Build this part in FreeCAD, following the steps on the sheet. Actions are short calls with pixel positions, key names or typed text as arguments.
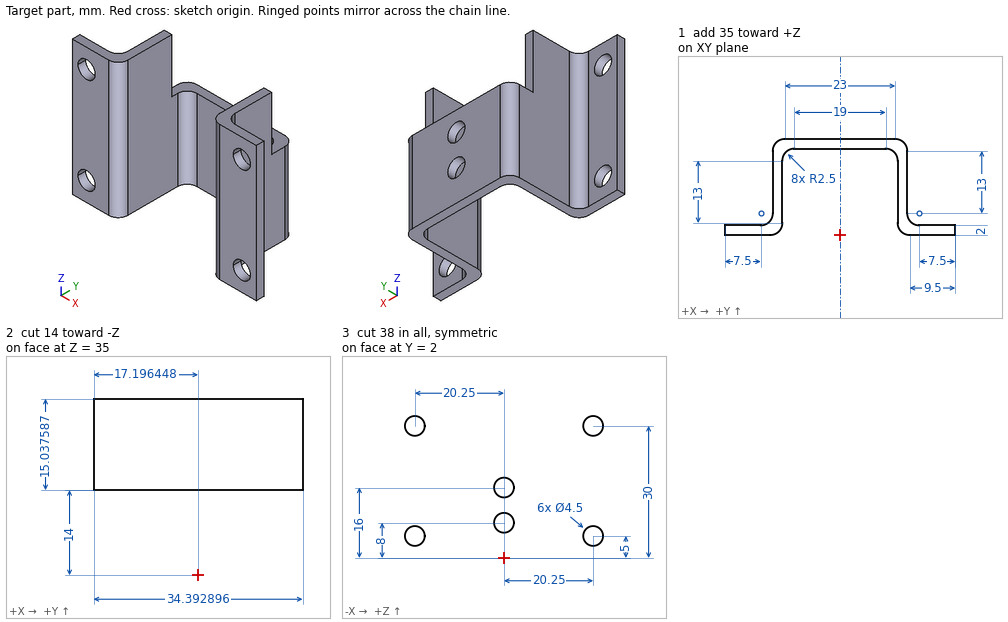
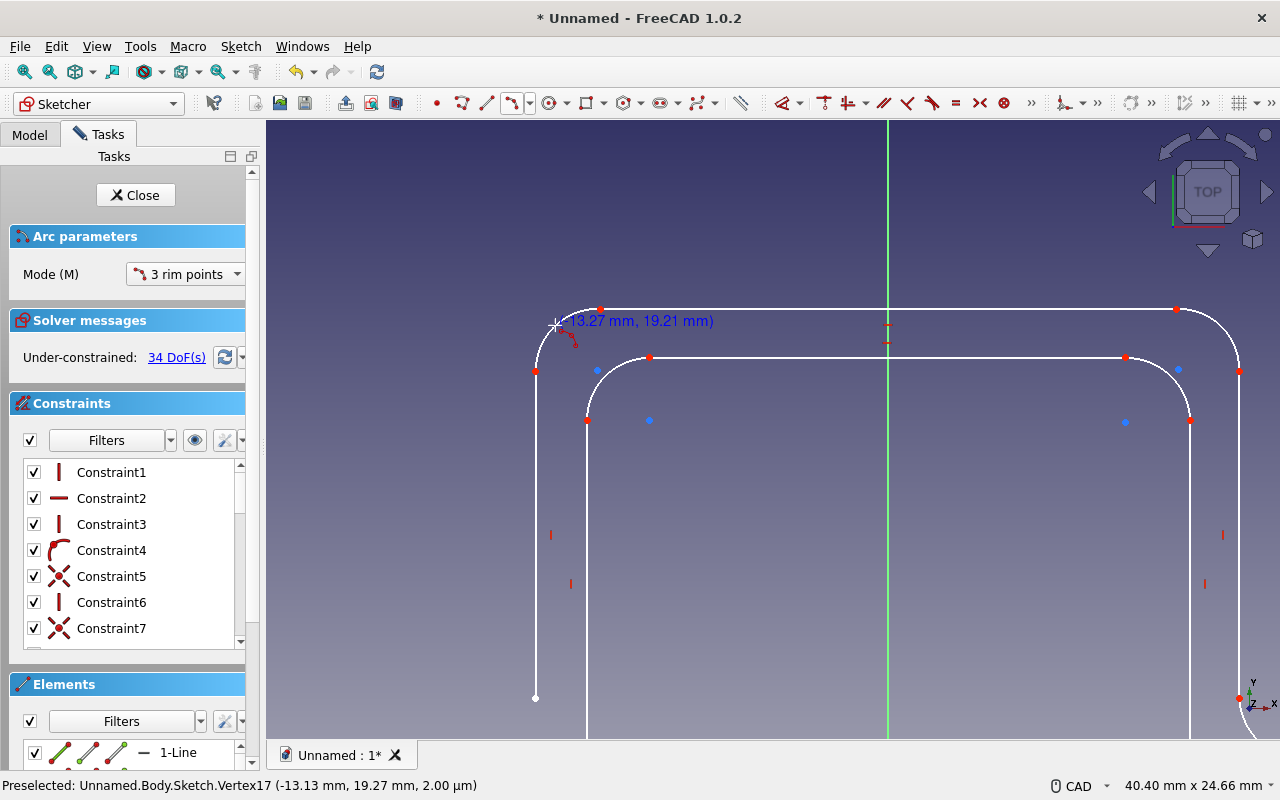
click(536, 698)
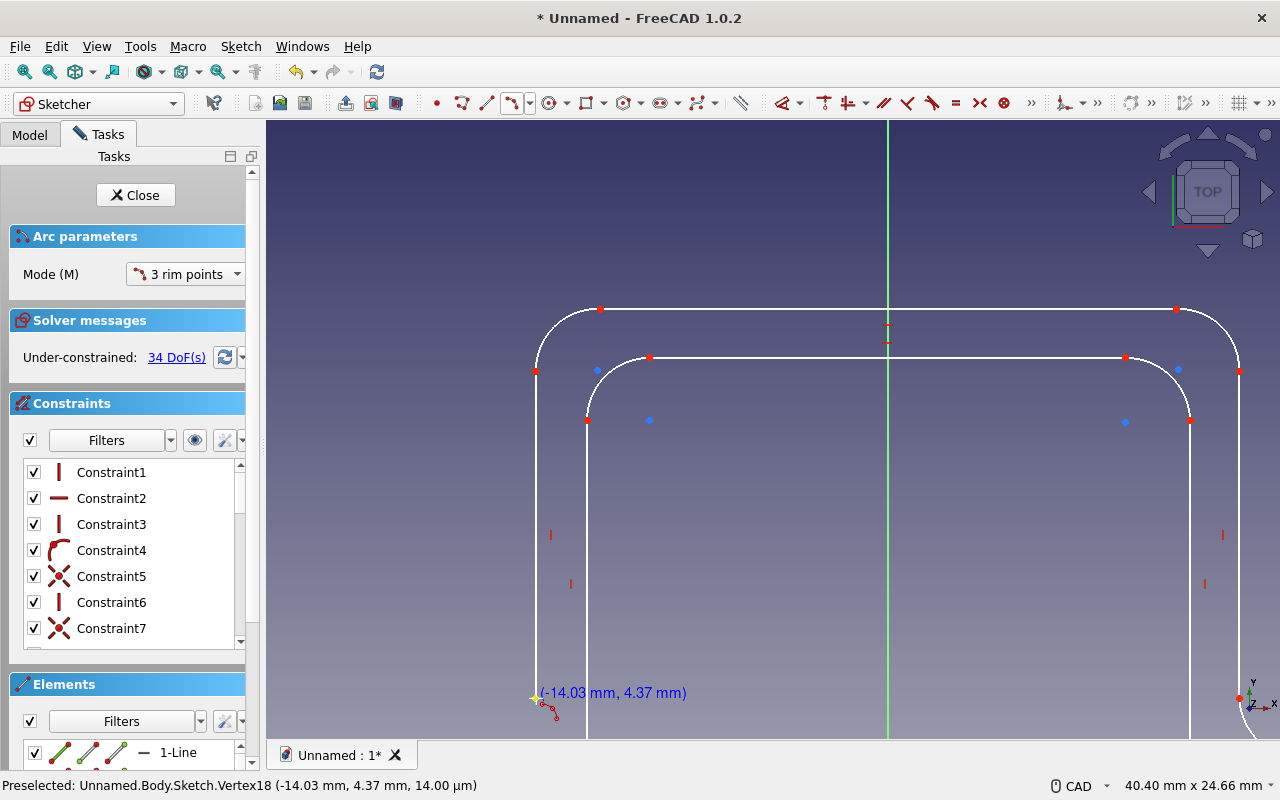
scroll(555, 325, down, 4)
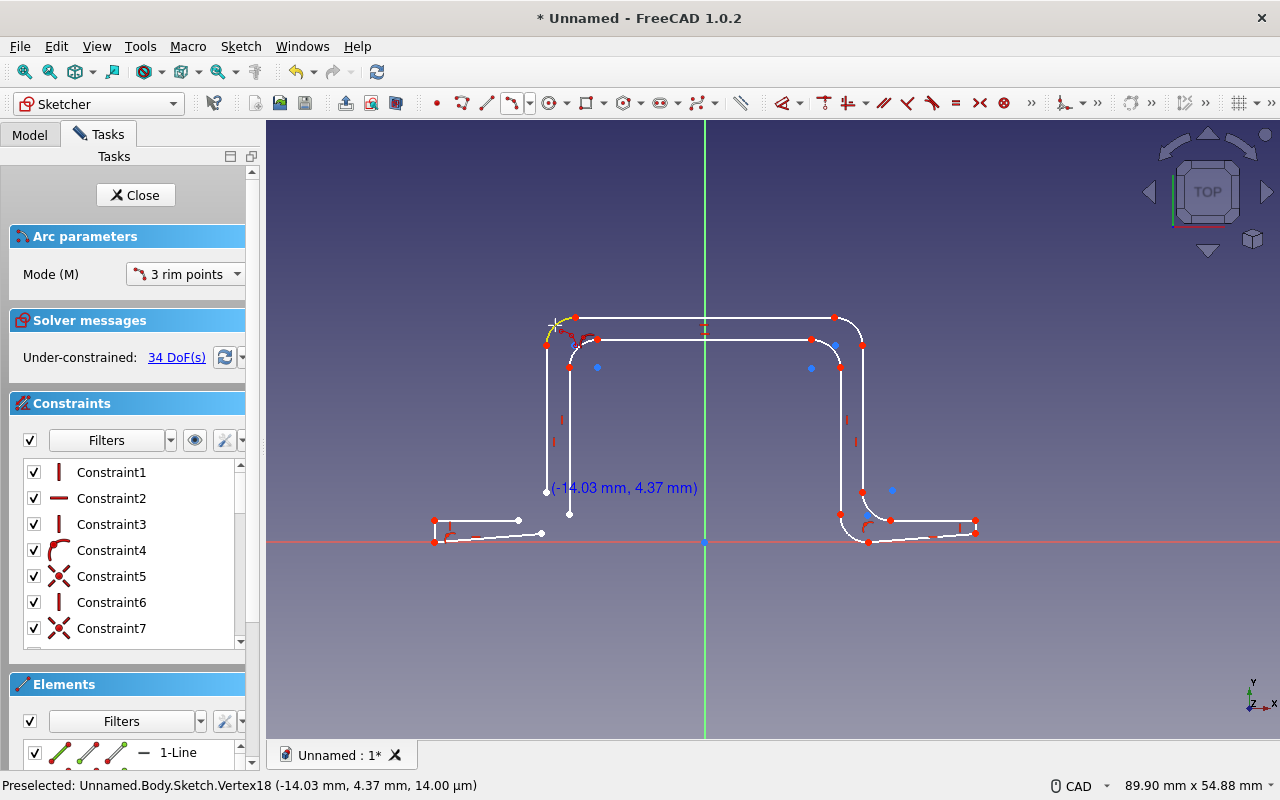
click(519, 521)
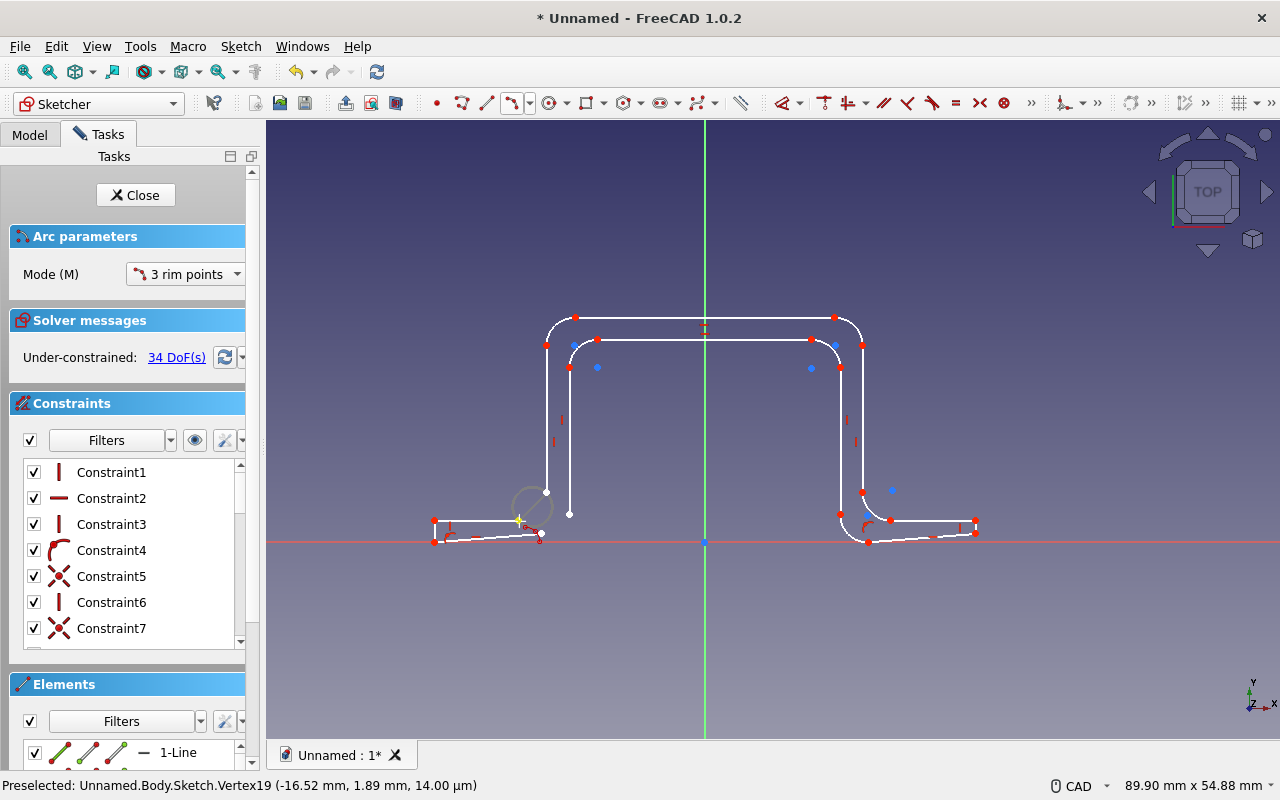
scroll(539, 511, up, 4)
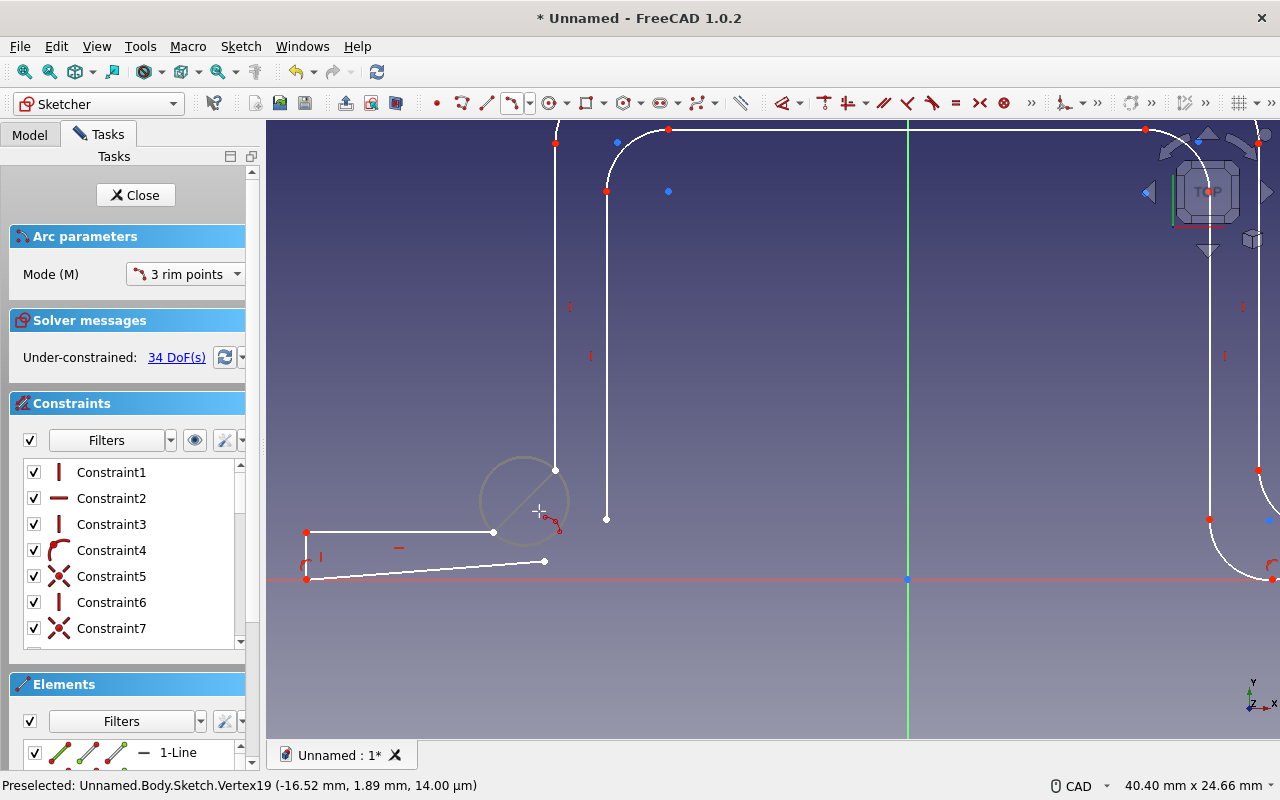
click(538, 511)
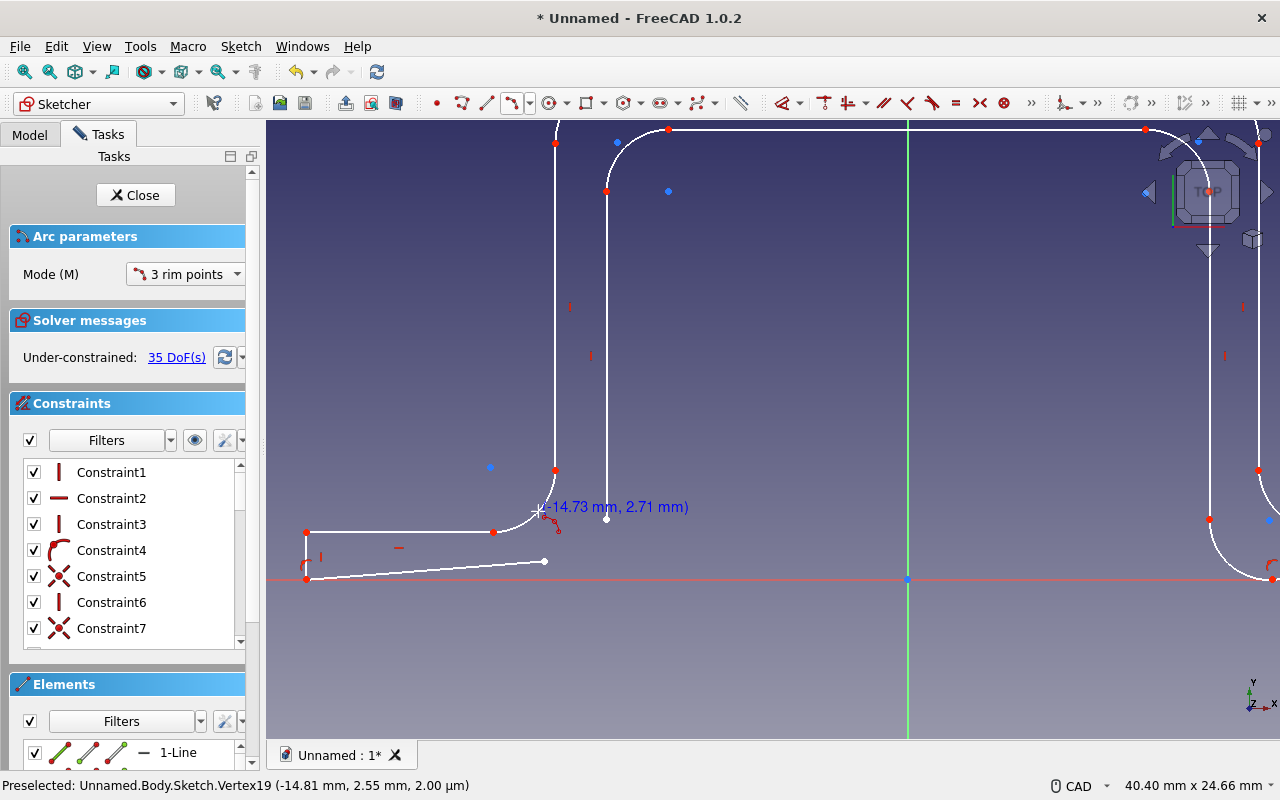
click(544, 561)
click(607, 519)
click(588, 562)
key(Escape)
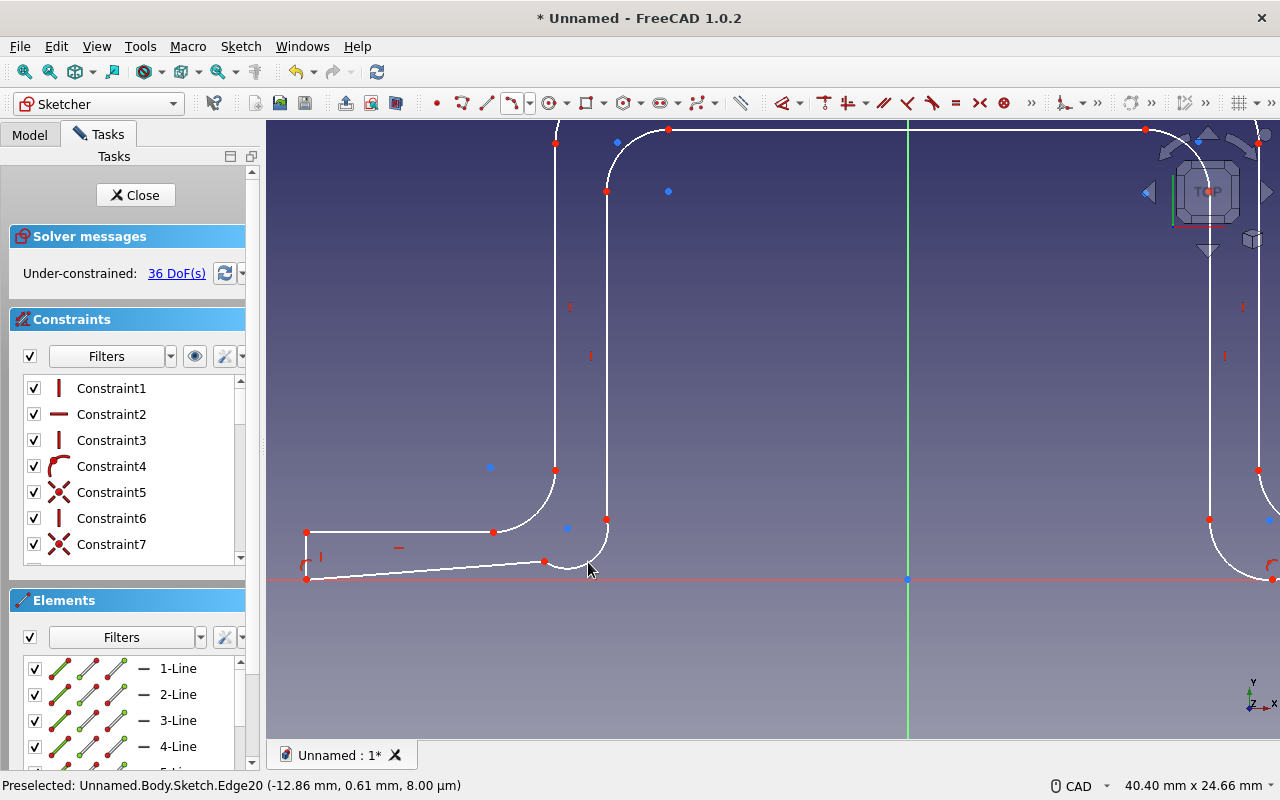
click(607, 421)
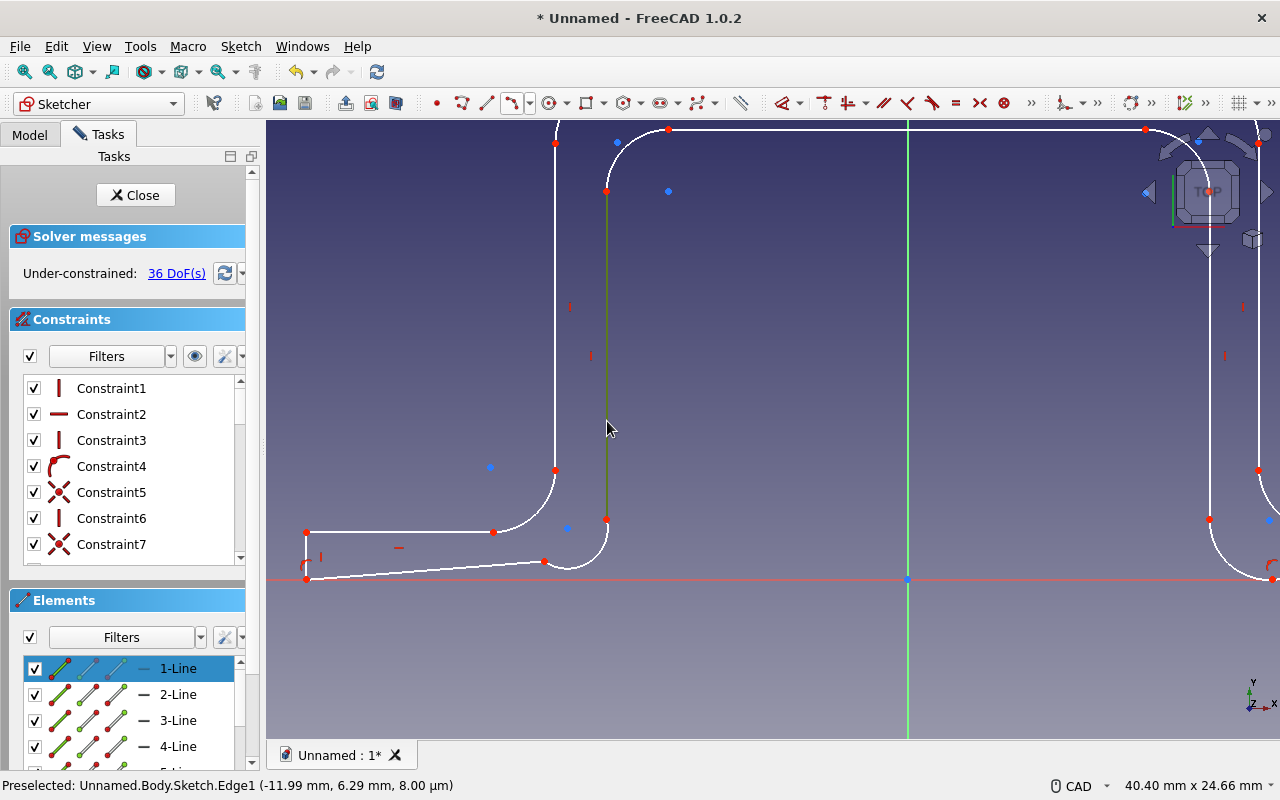
click(613, 164)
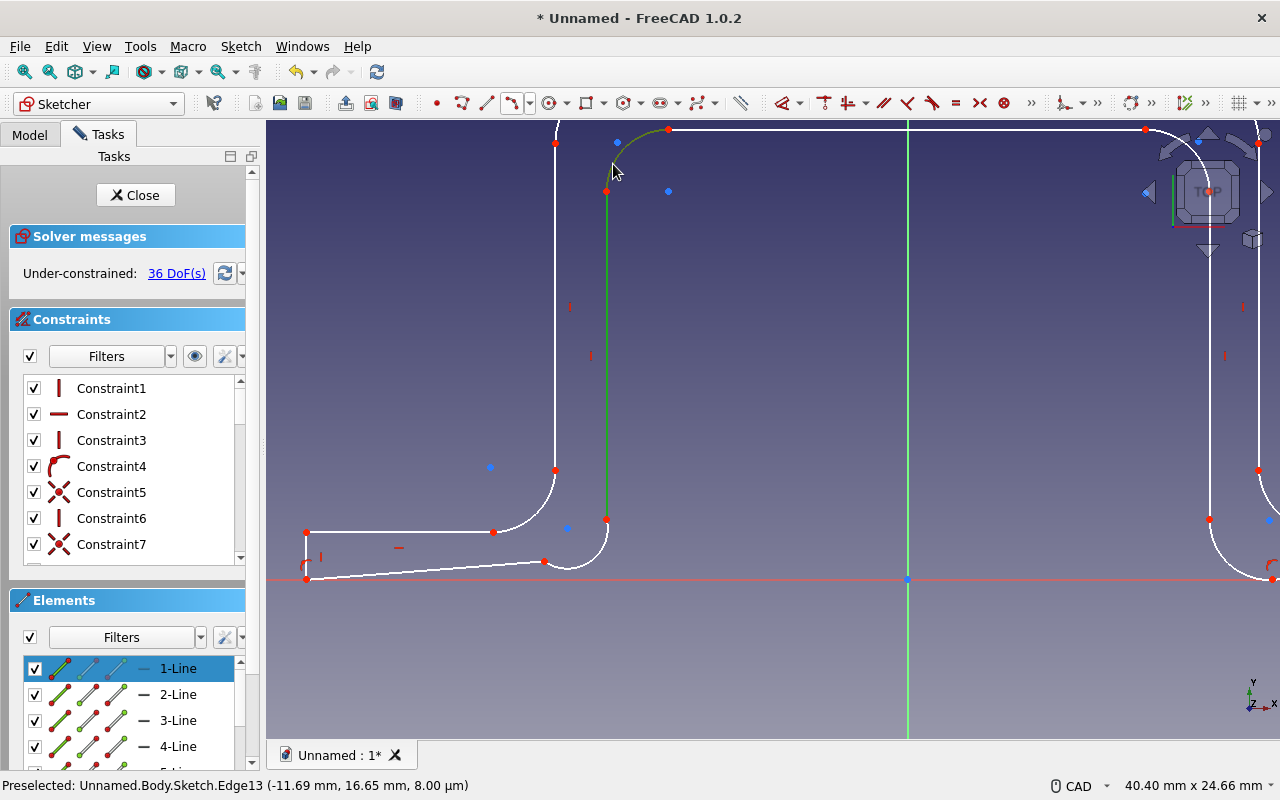
click(932, 104)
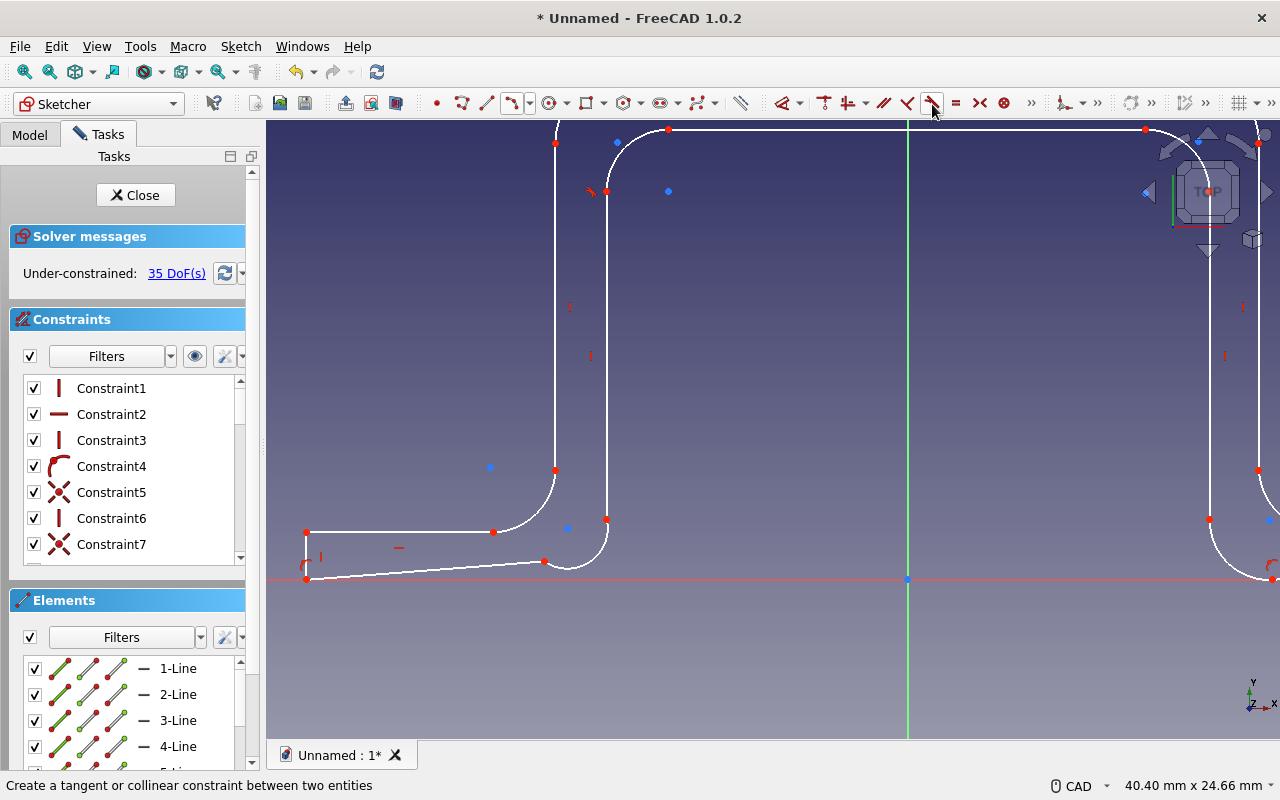
click(607, 421)